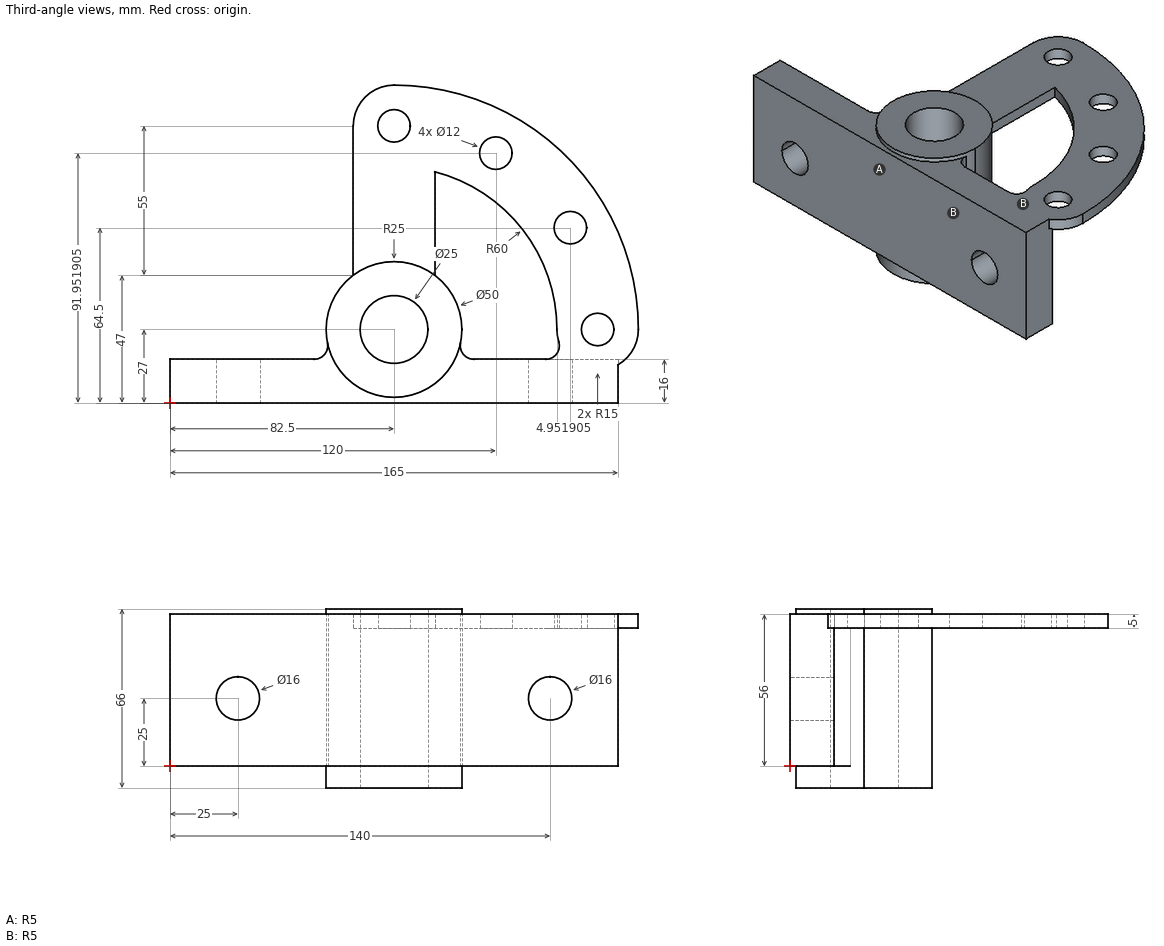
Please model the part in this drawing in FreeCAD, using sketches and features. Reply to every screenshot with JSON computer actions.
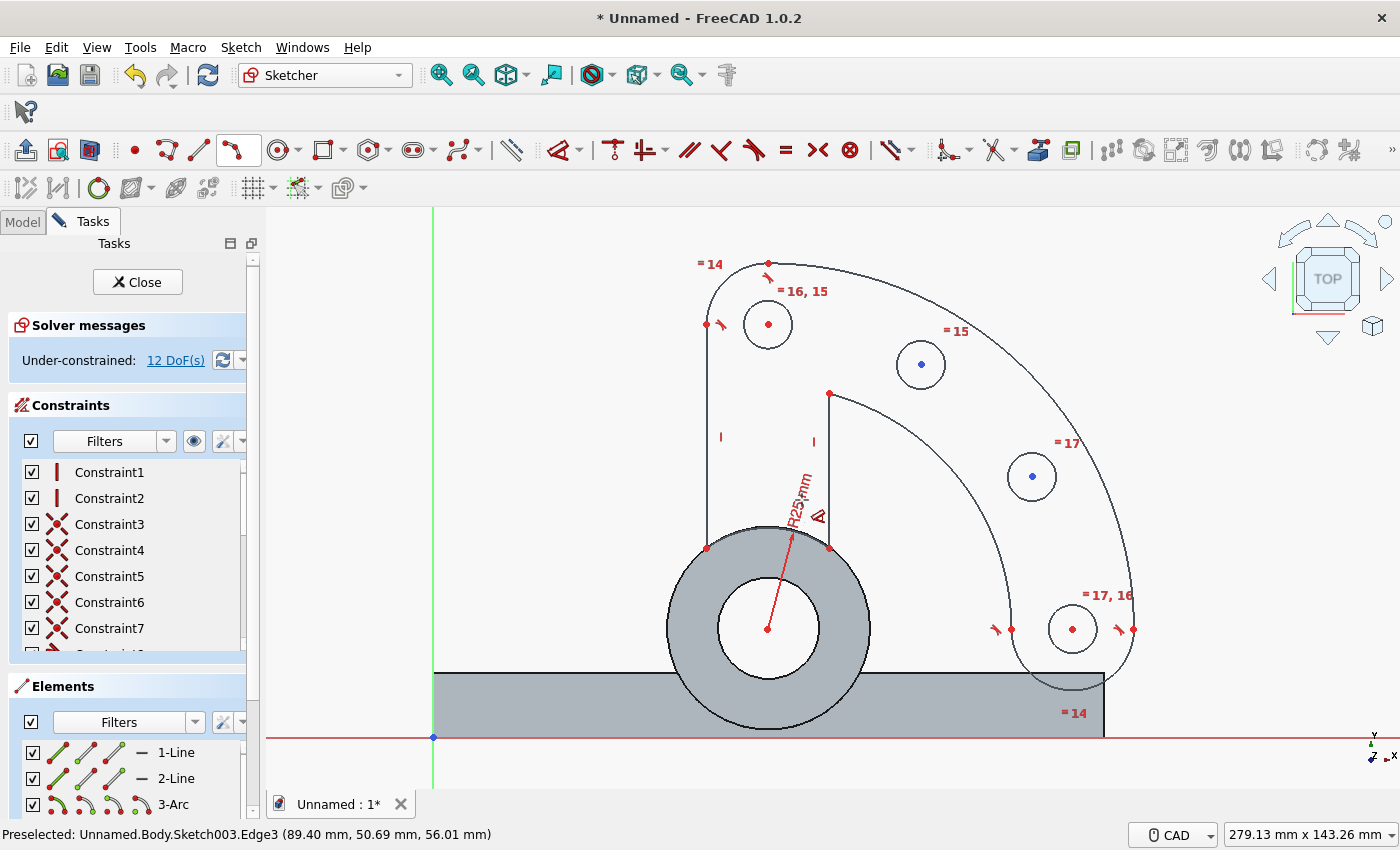
{"action": "left_click", "coordinate": [993, 536]}
{"action": "left_click", "coordinate": [1023, 524]}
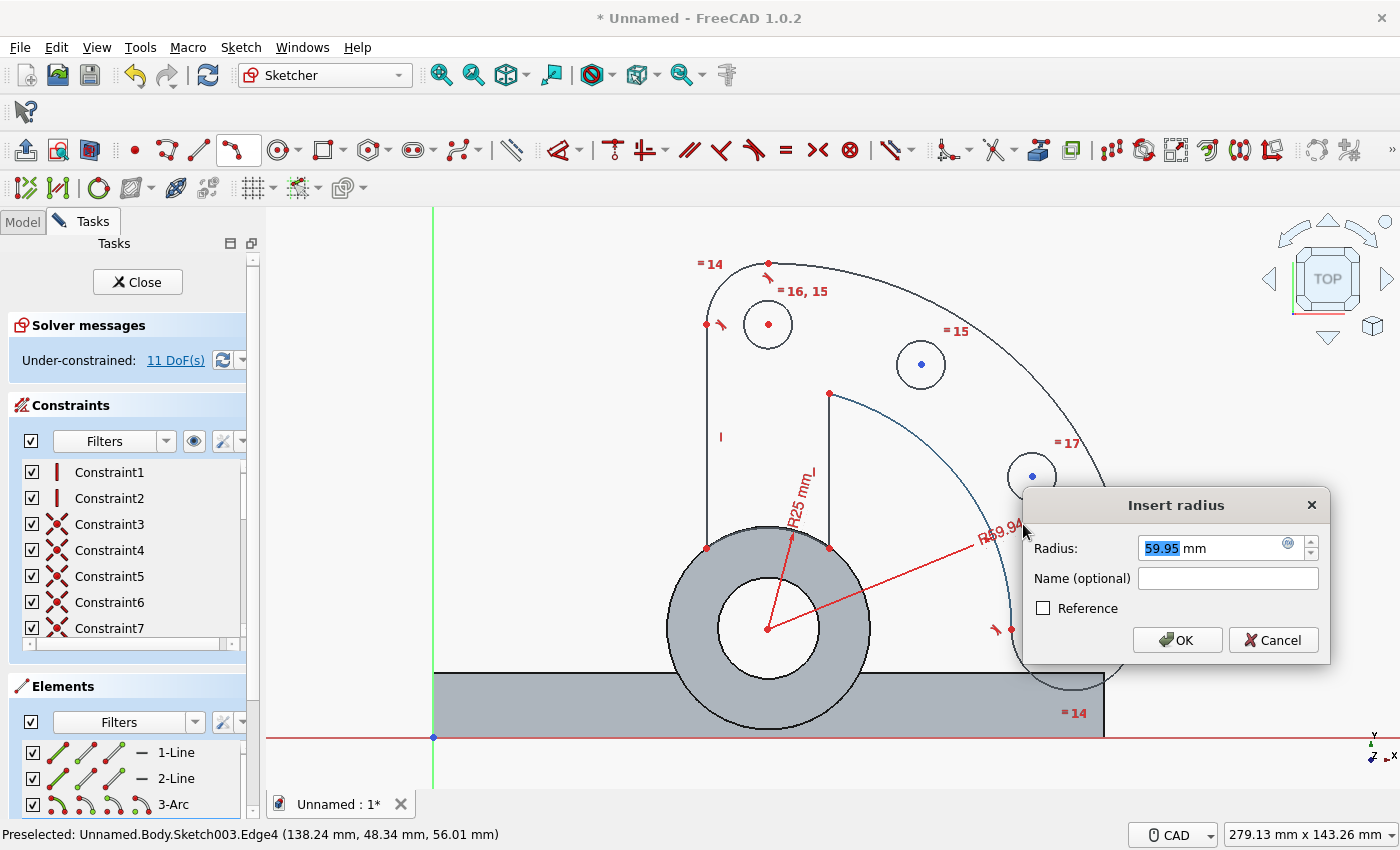
{"action": "type", "text": "60"}
{"action": "key", "text": "Return"}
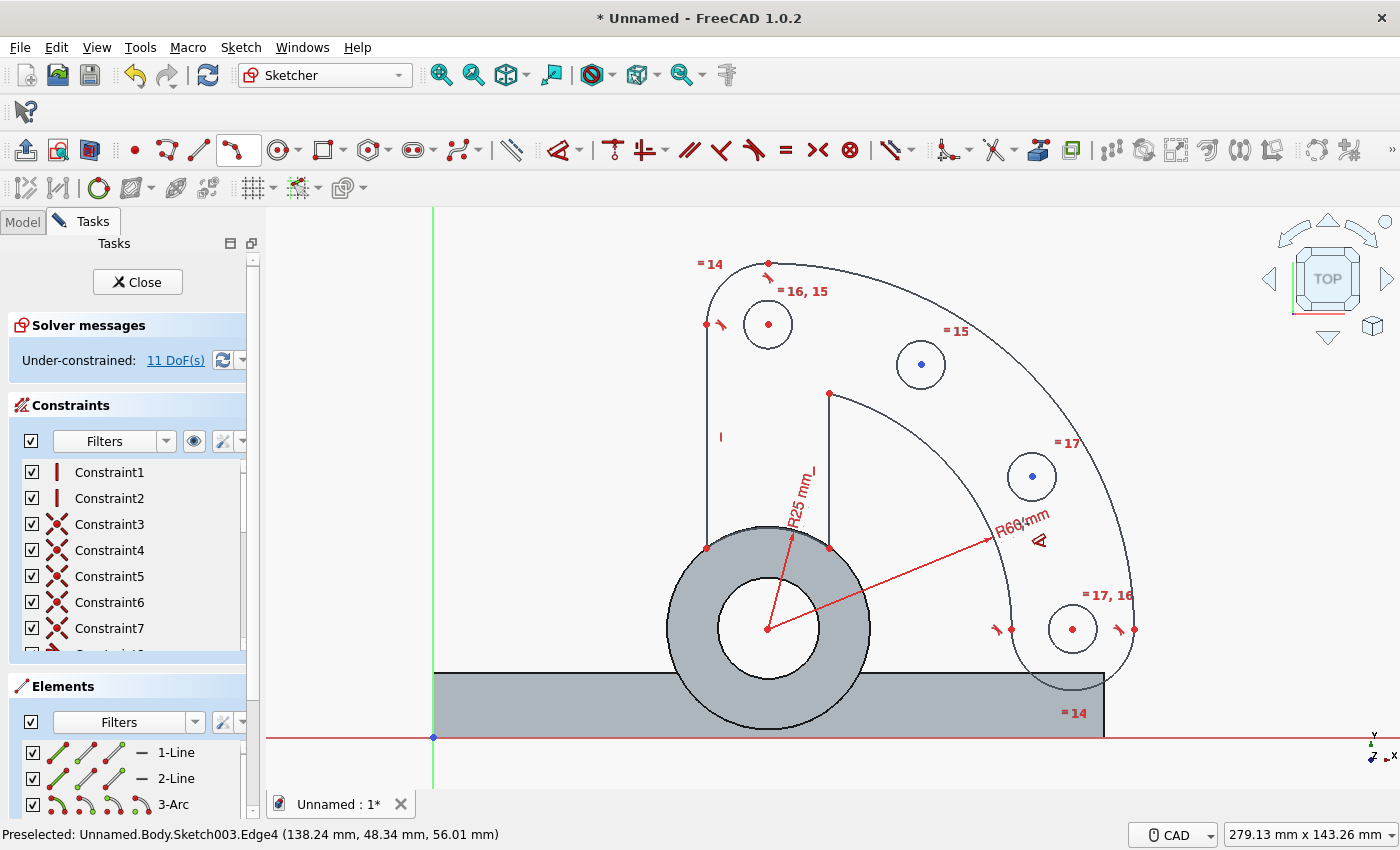
{"action": "left_click", "coordinate": [1037, 679]}
{"action": "left_click", "coordinate": [1018, 705]}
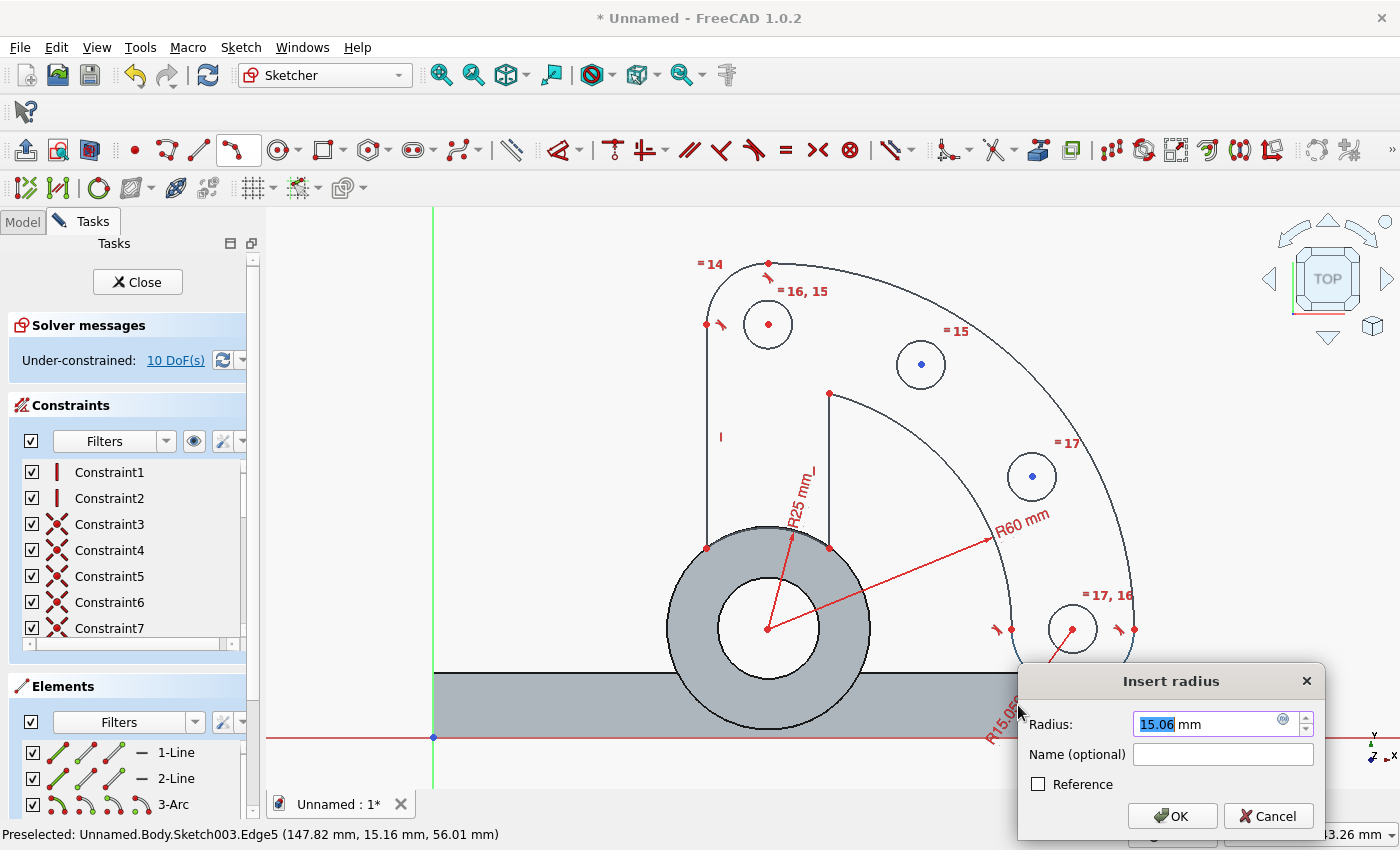
{"action": "type", "text": "15"}
{"action": "key", "text": "Return"}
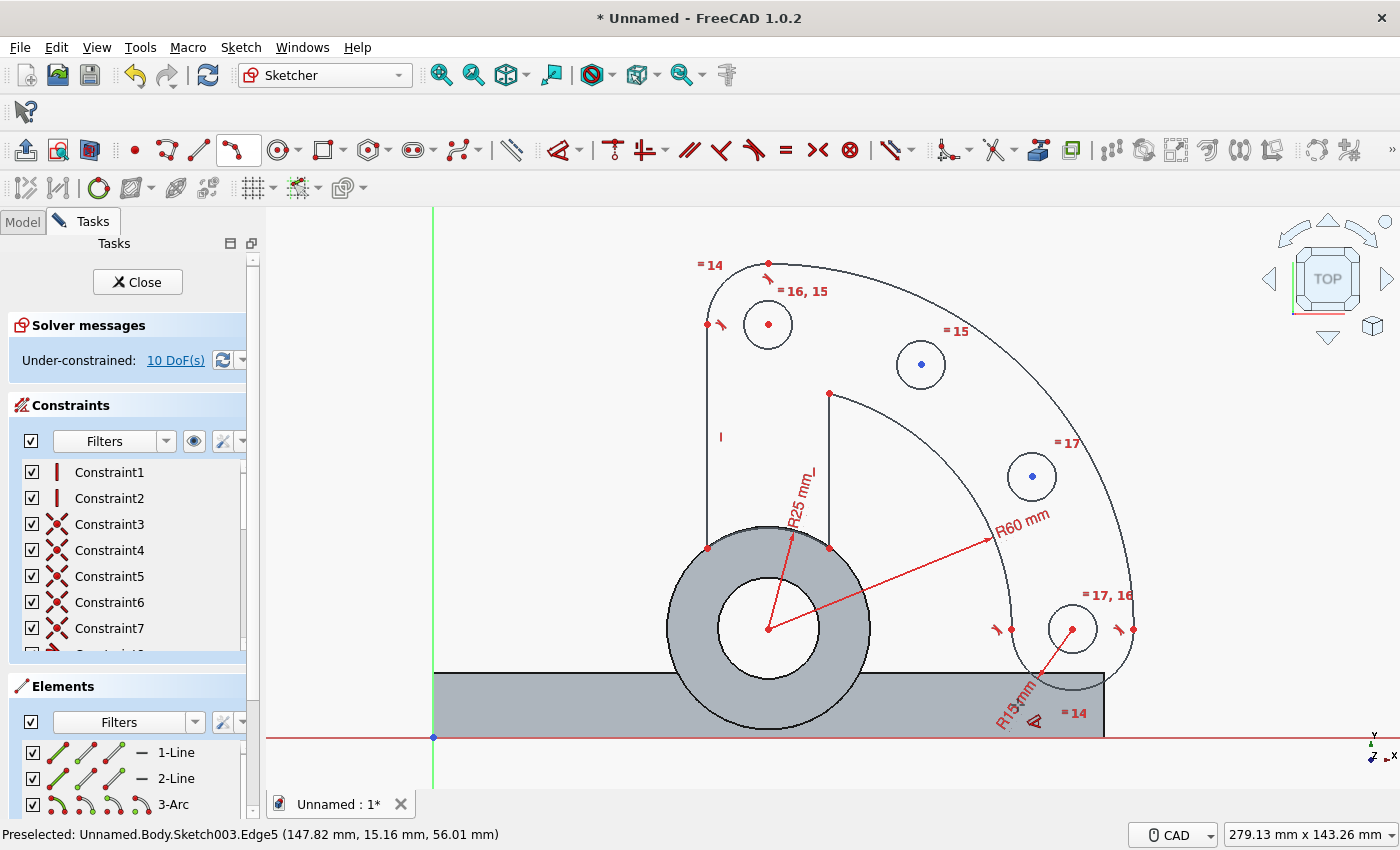
{"action": "left_click", "coordinate": [938, 348]}
{"action": "left_click", "coordinate": [975, 349]}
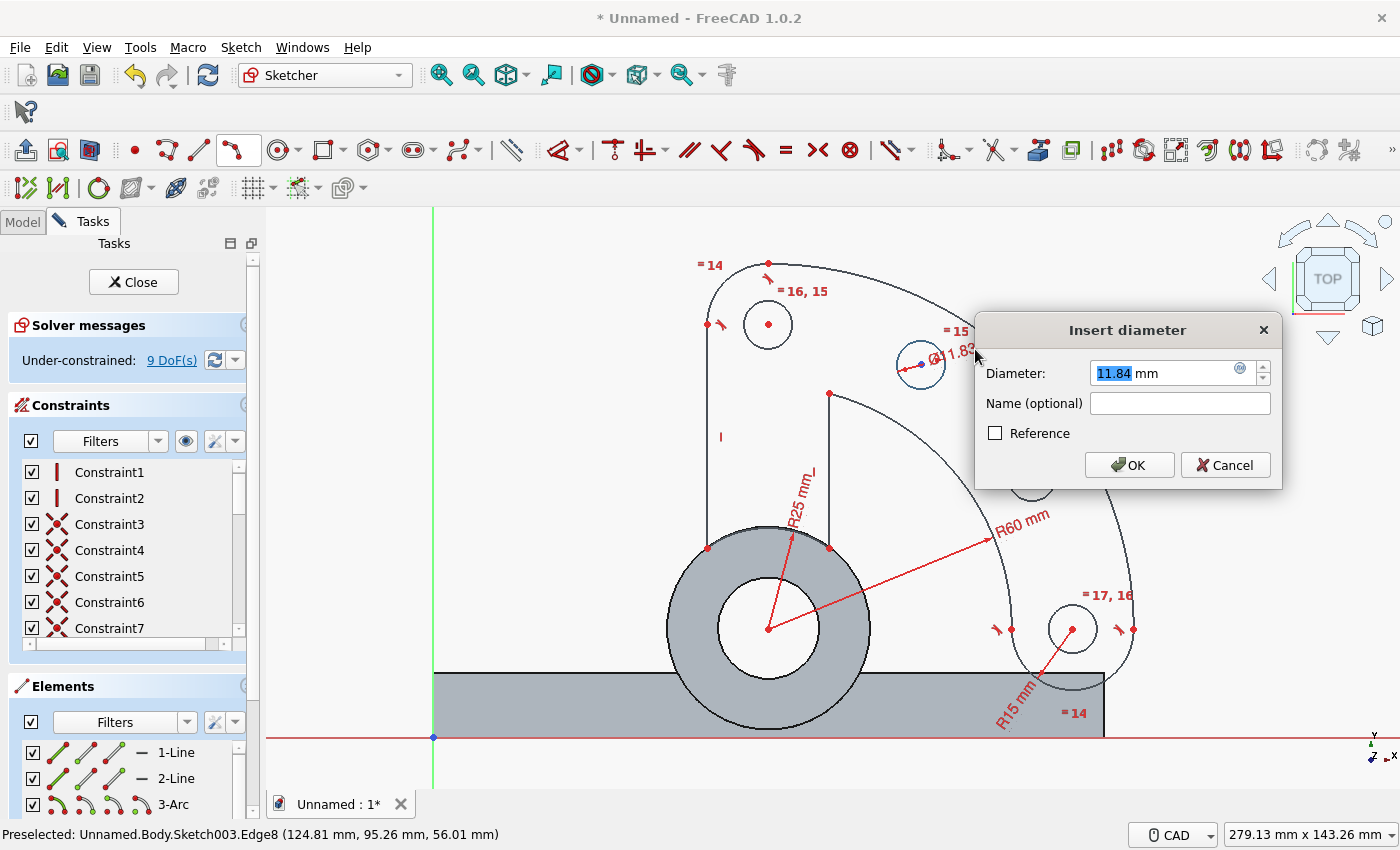
{"action": "type", "text": "12"}
{"action": "key", "text": "Return"}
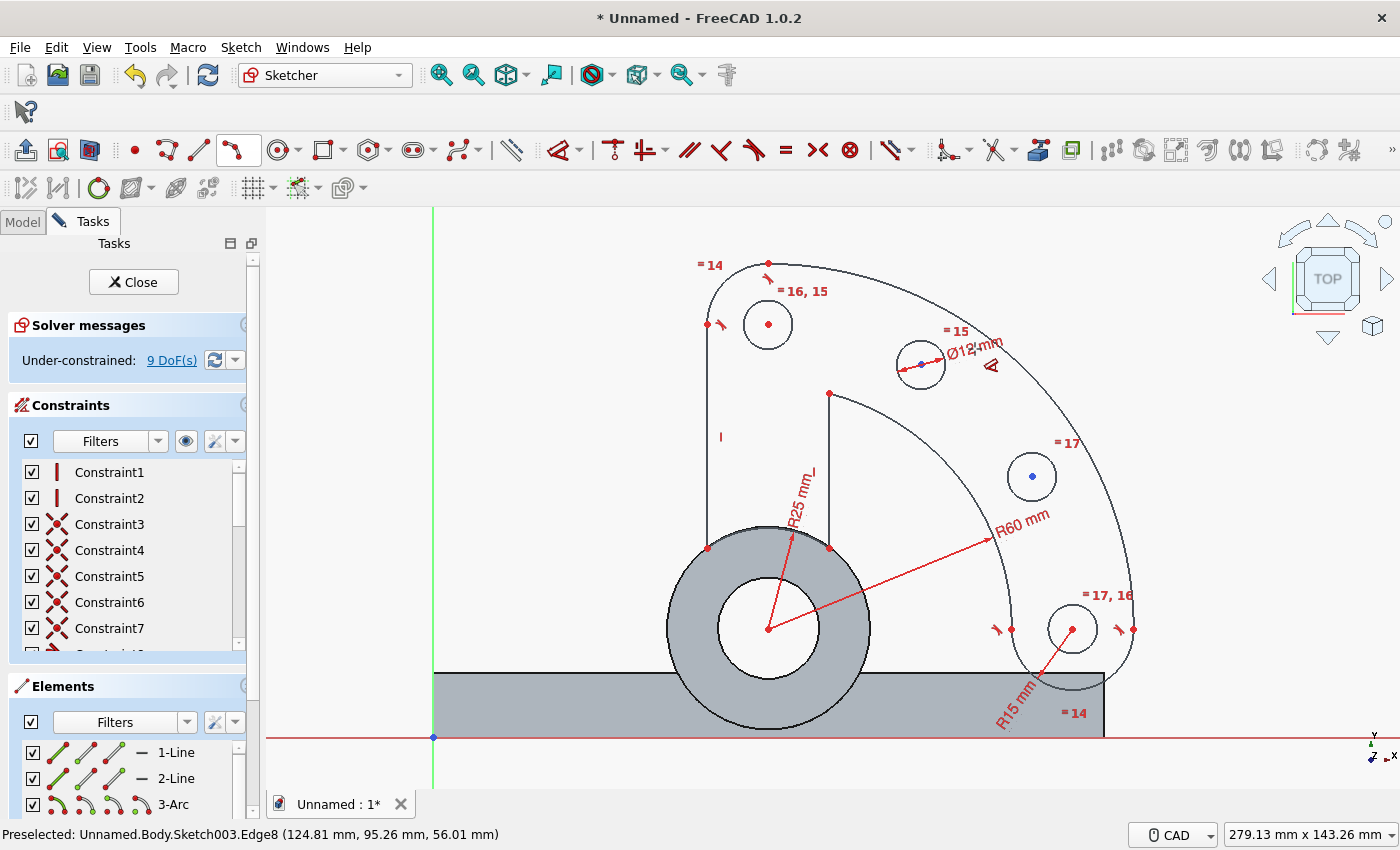
{"action": "left_click", "coordinate": [707, 392]}
{"action": "left_click", "coordinate": [673, 437]}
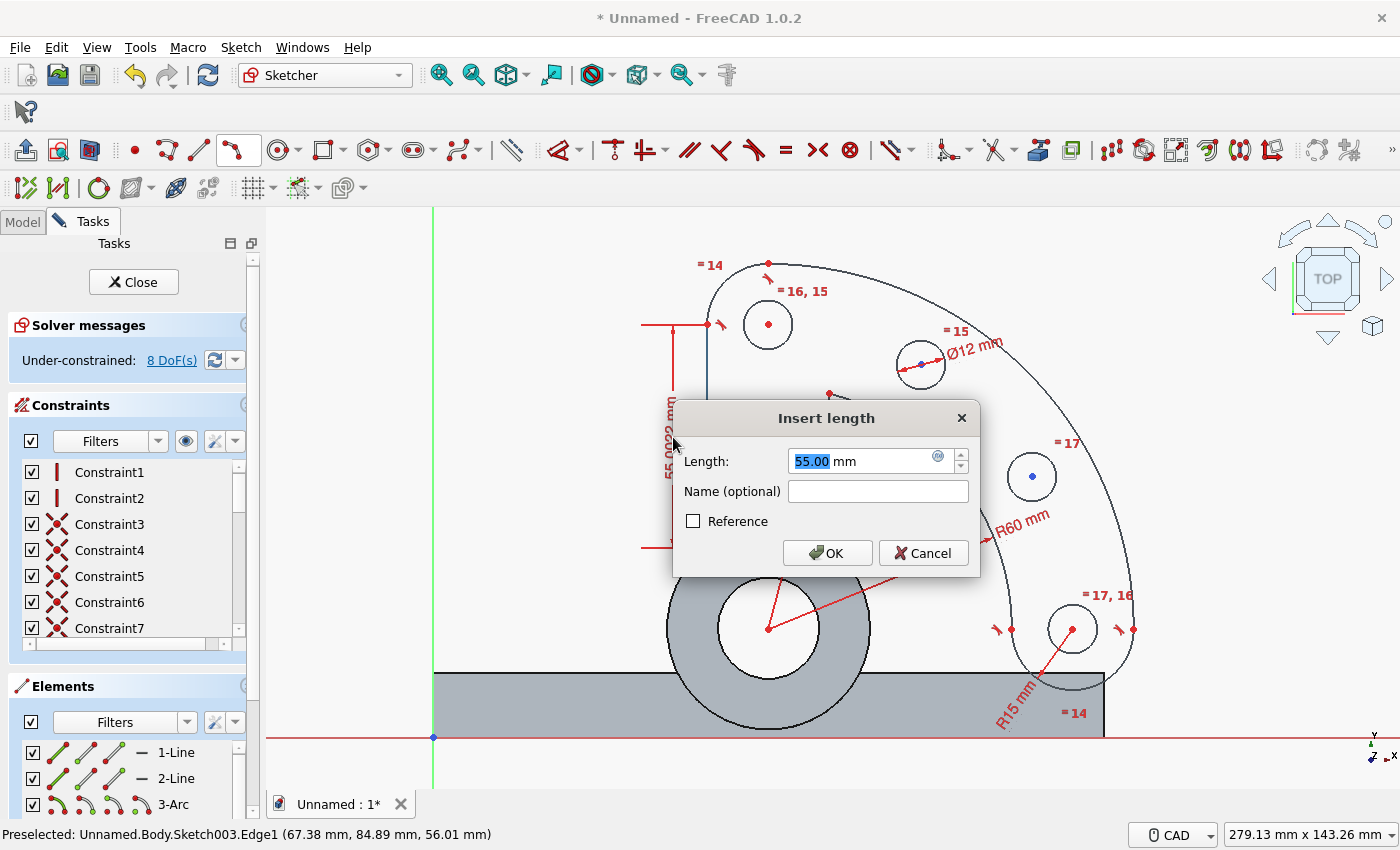
{"action": "type", "text": "55"}
{"action": "key", "text": "Return"}